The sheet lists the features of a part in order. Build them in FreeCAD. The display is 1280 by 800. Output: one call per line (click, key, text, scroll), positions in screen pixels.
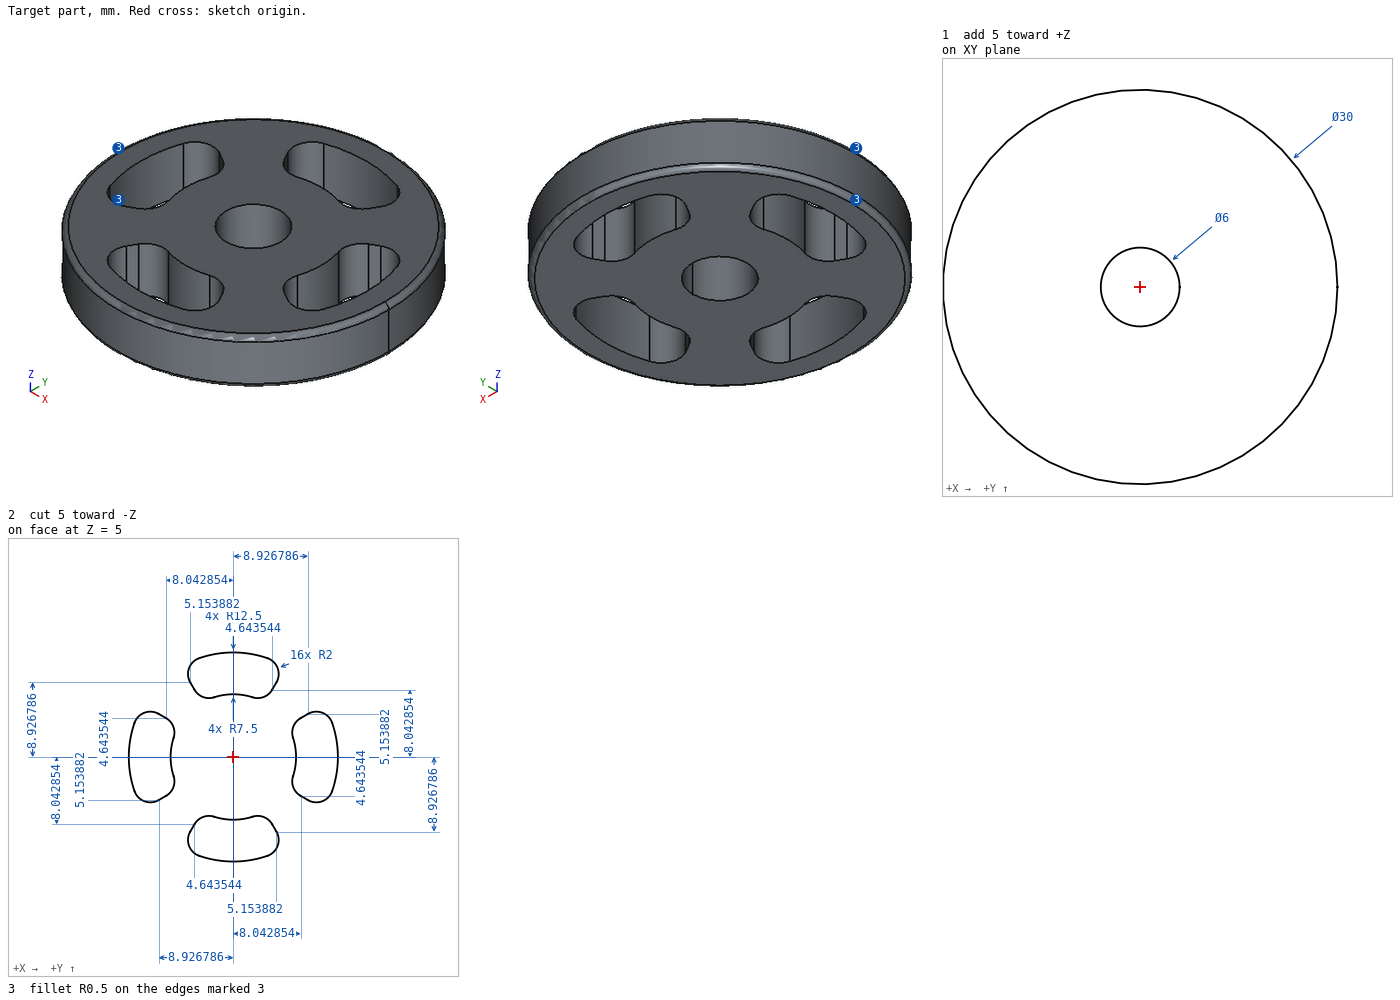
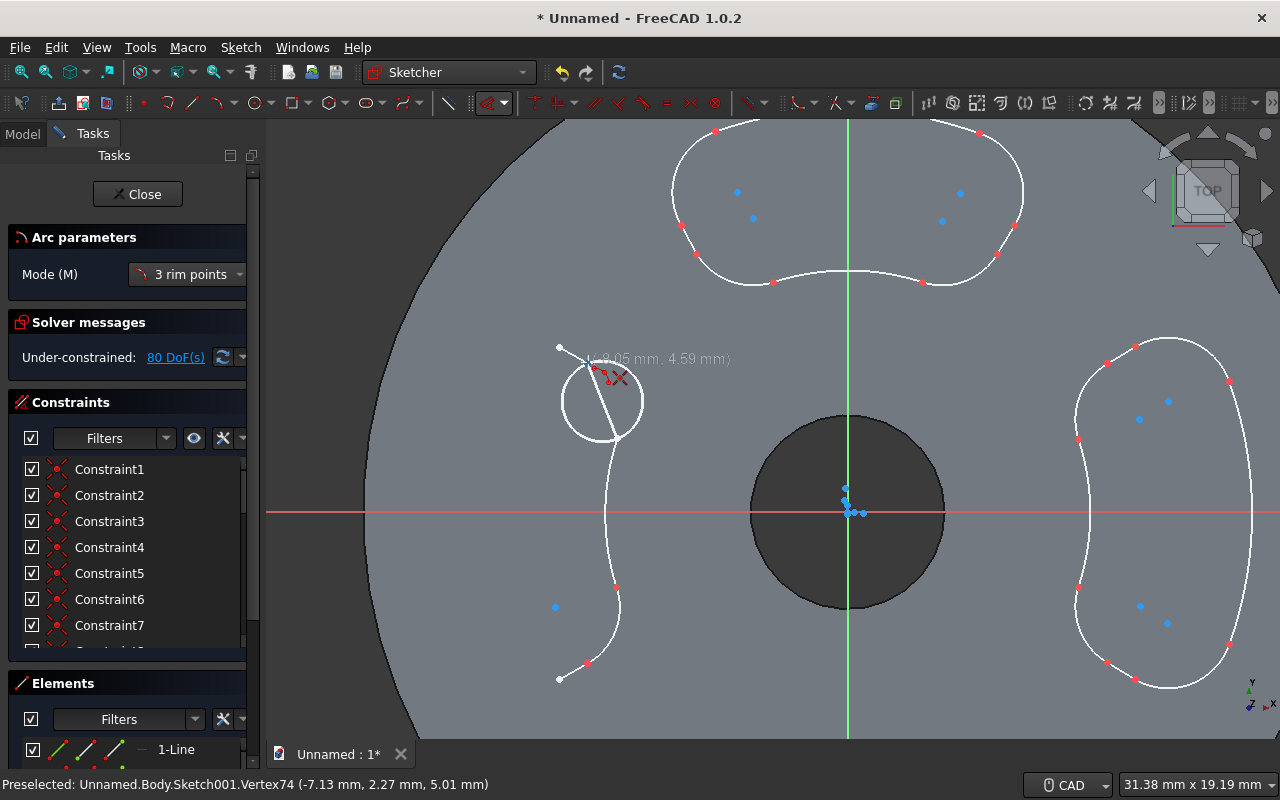
click(587, 363)
click(616, 395)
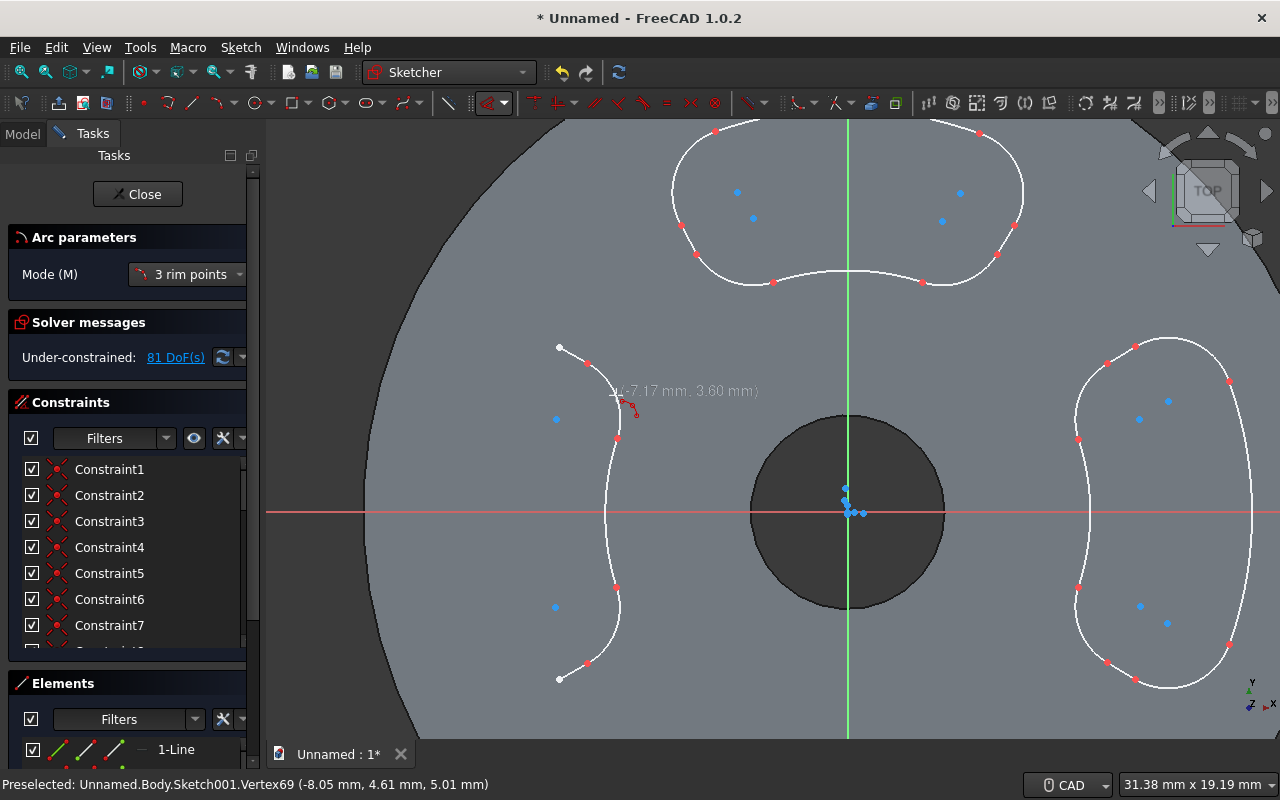
click(559, 347)
click(466, 381)
click(504, 341)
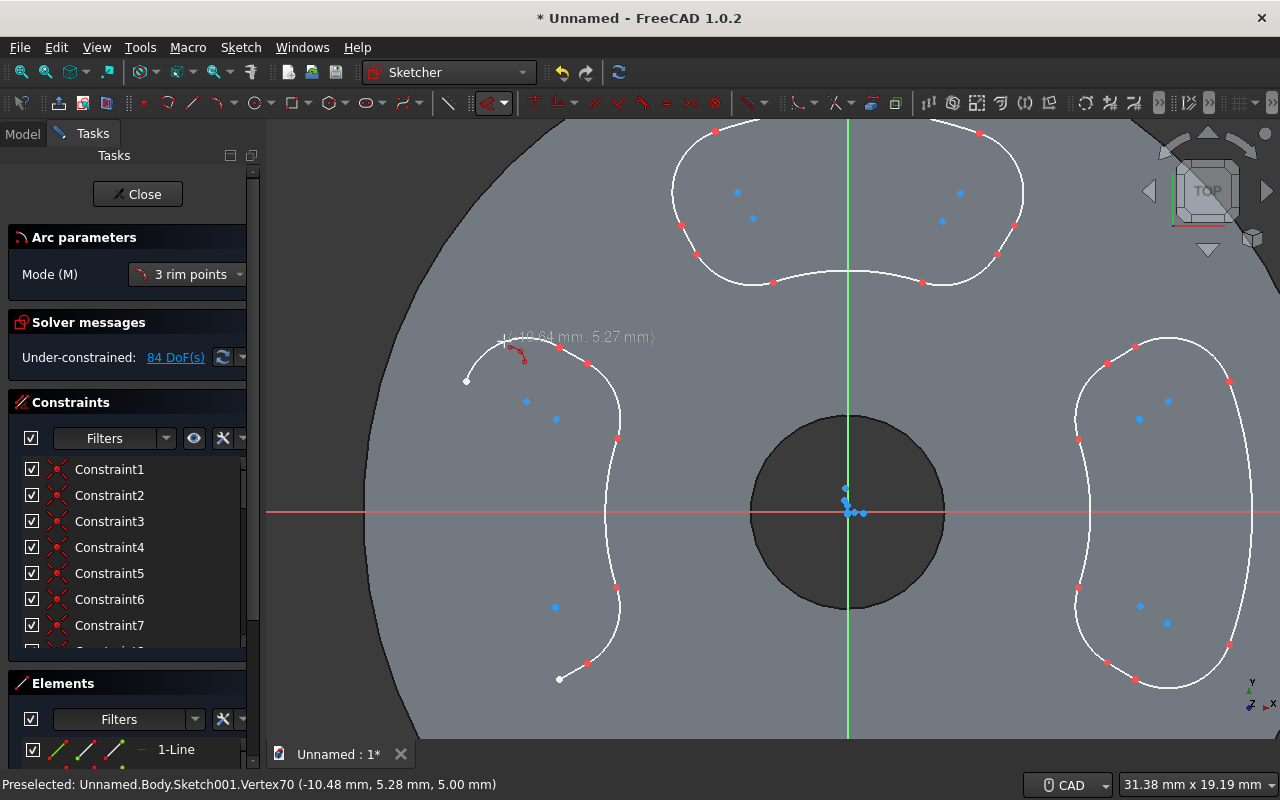
click(466, 382)
click(466, 644)
click(445, 485)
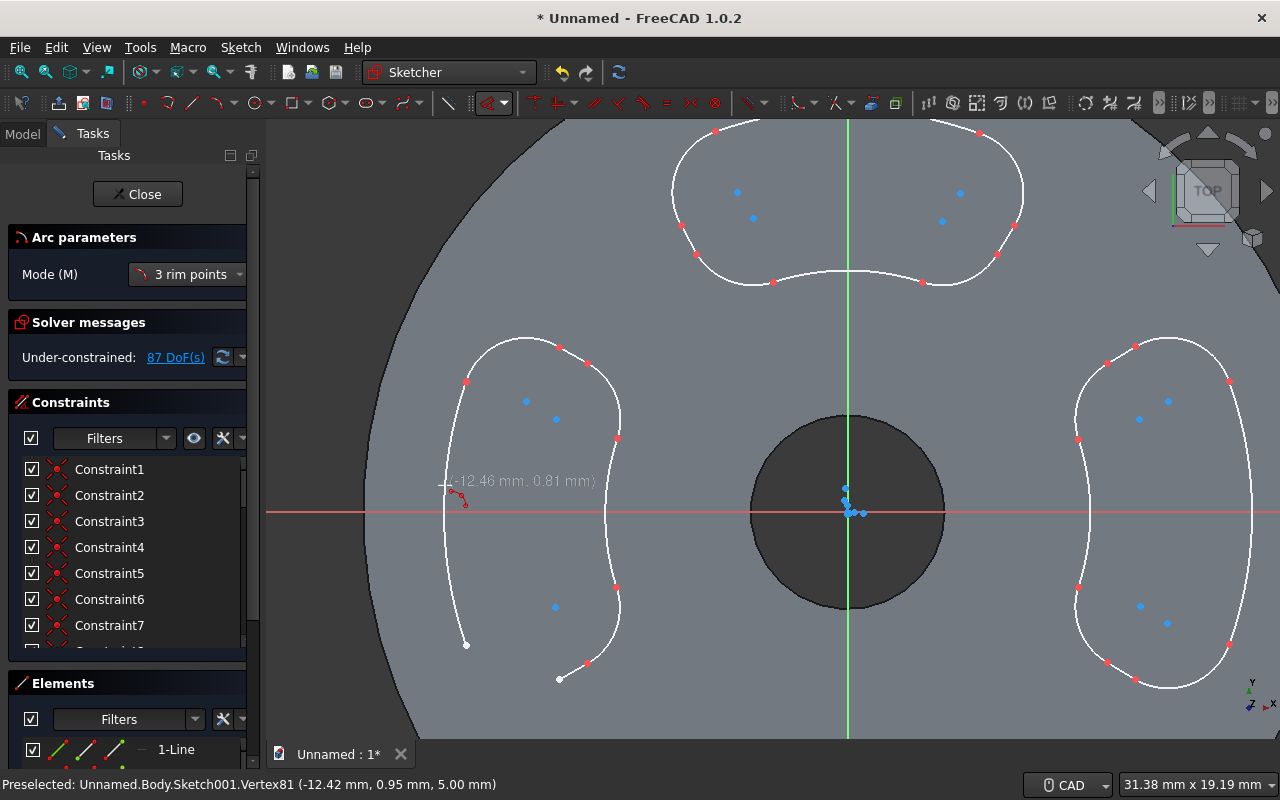
click(466, 645)
click(559, 680)
click(504, 683)
key(Escape)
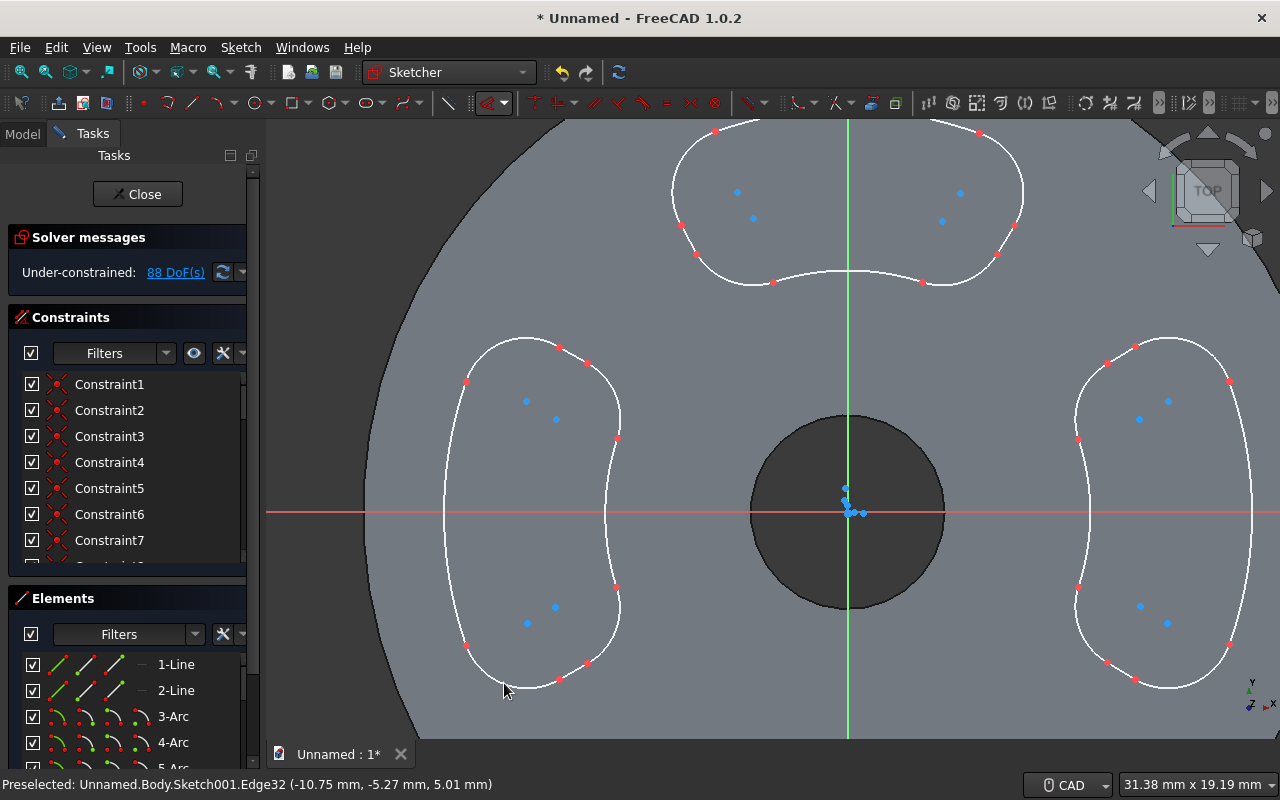
scroll(686, 234, up, 2)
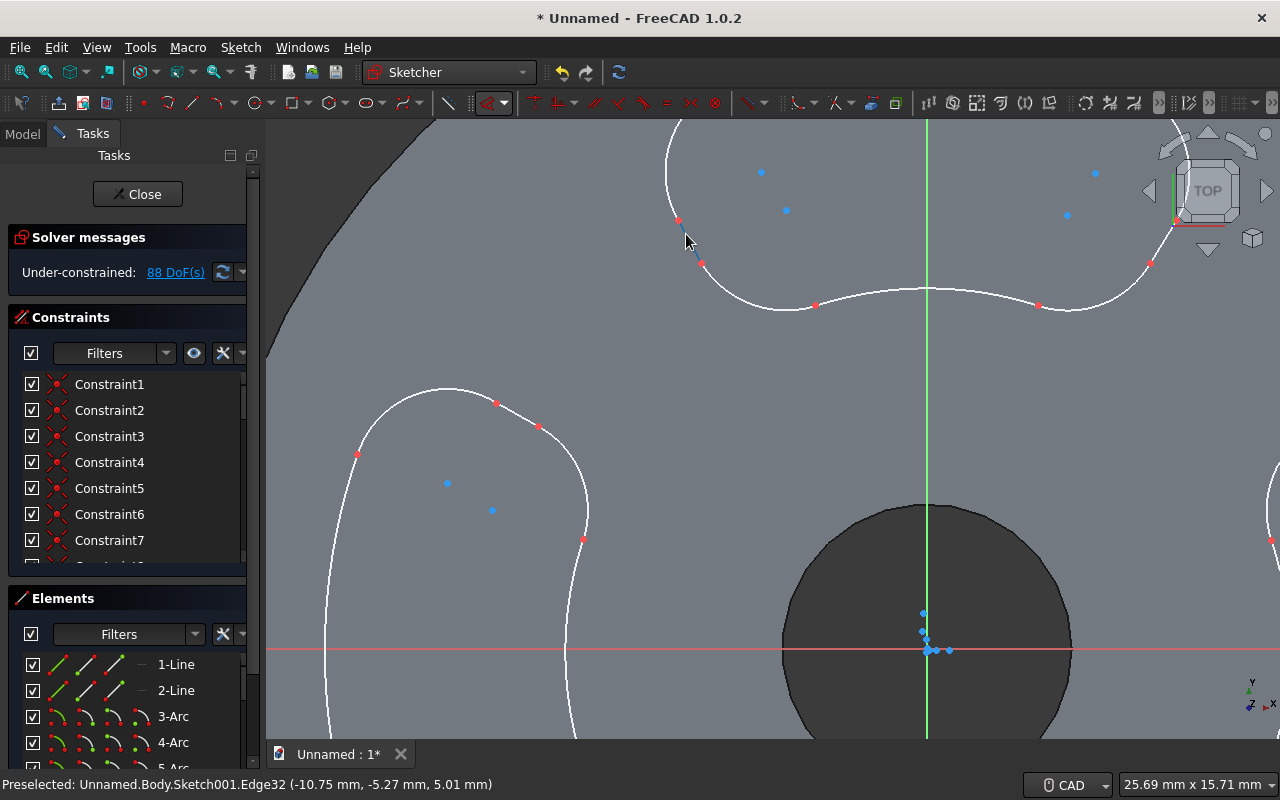
click(686, 234)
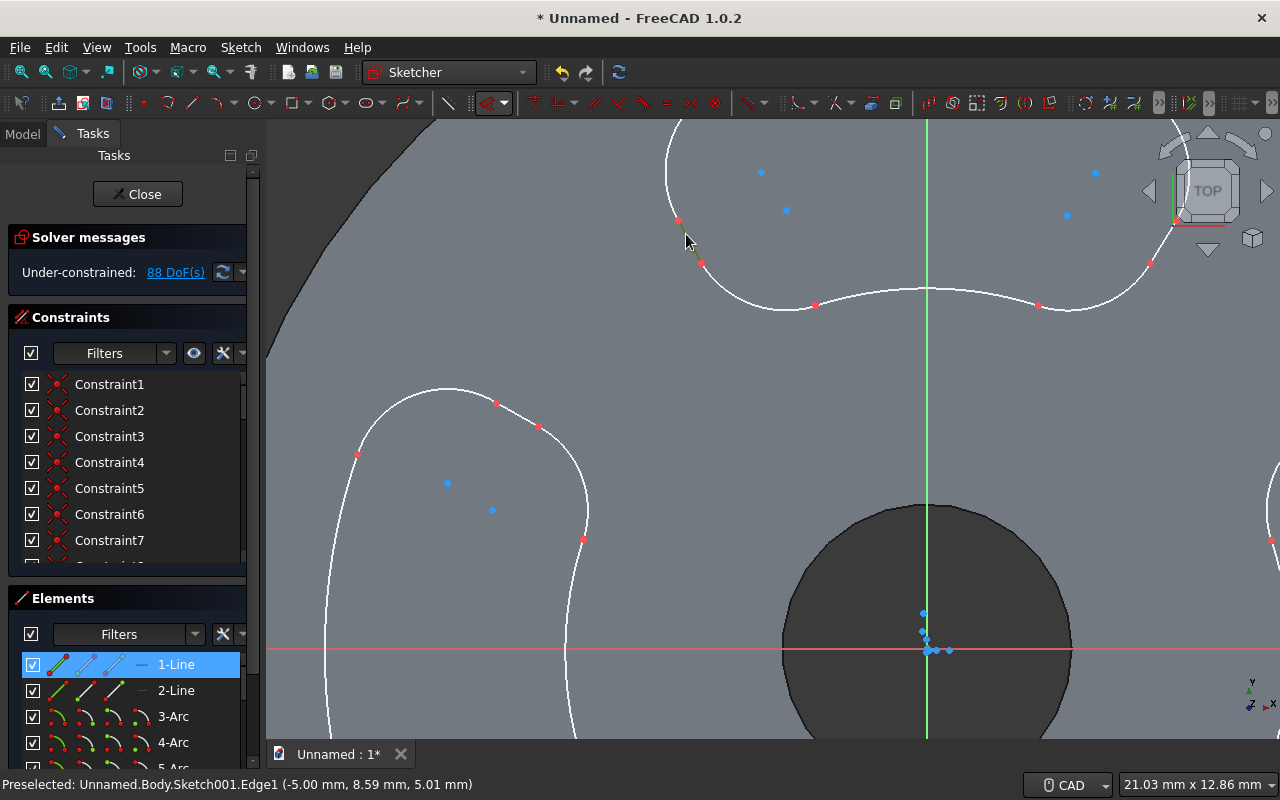
click(729, 292)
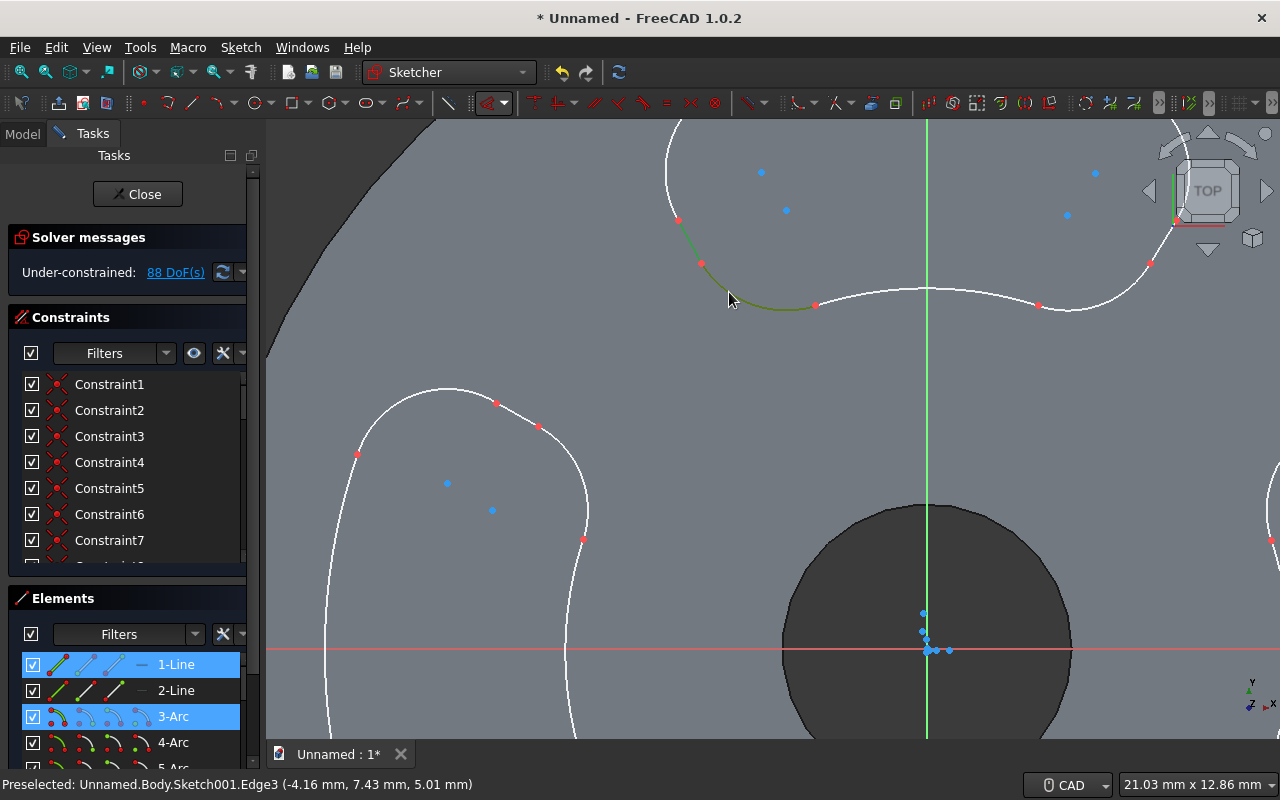
click(644, 104)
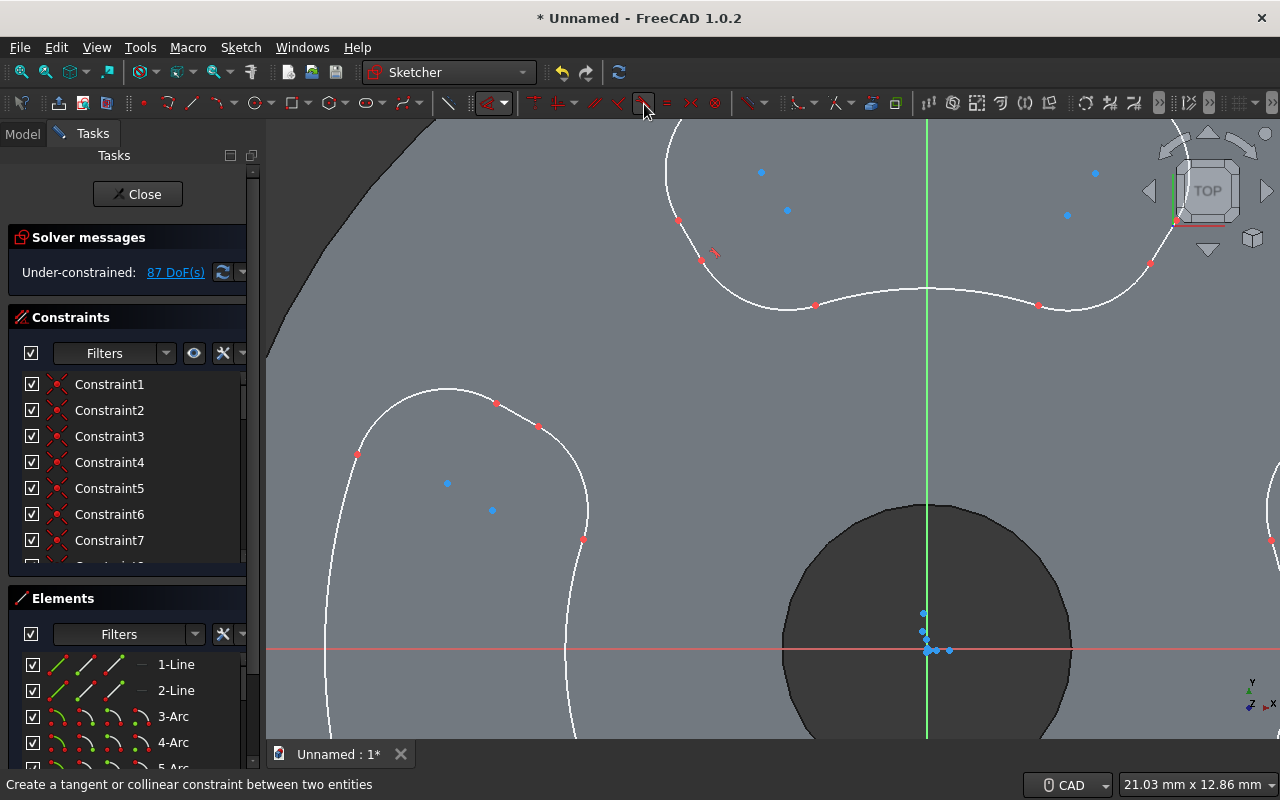
click(686, 233)